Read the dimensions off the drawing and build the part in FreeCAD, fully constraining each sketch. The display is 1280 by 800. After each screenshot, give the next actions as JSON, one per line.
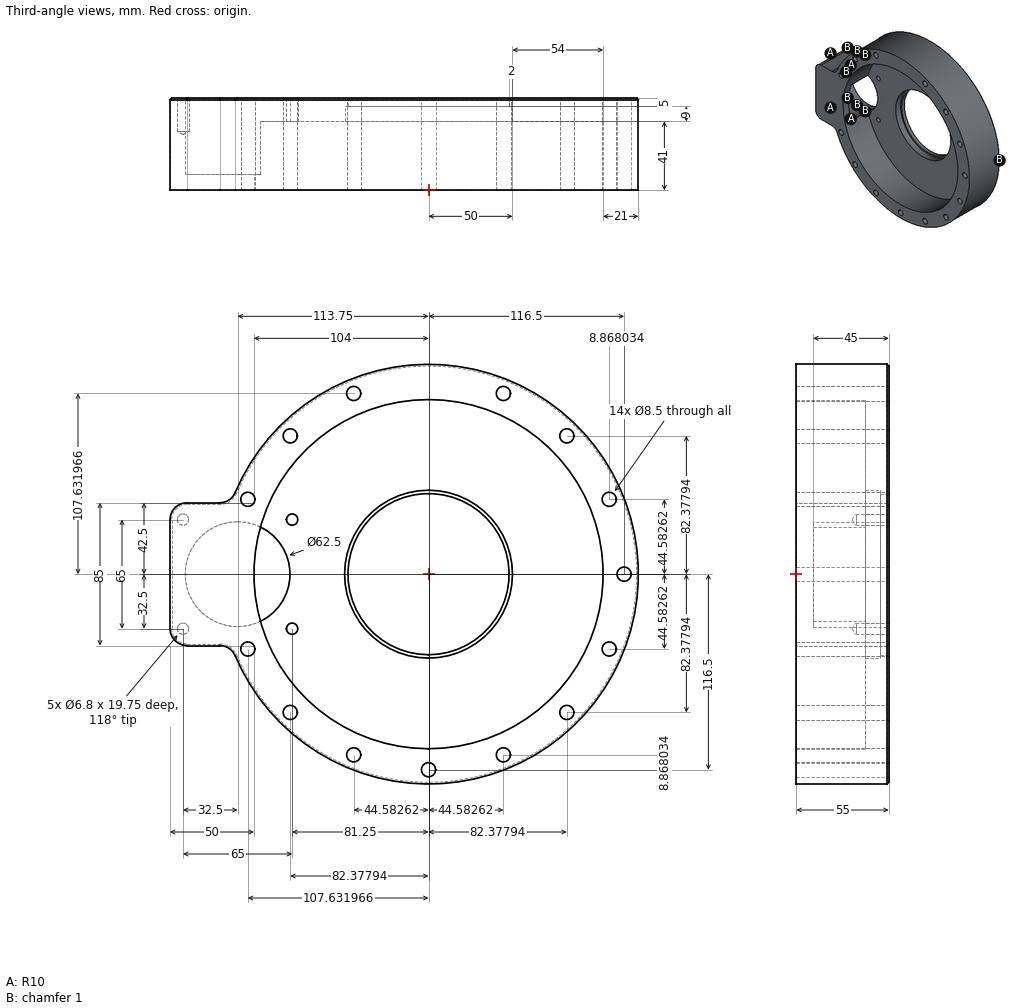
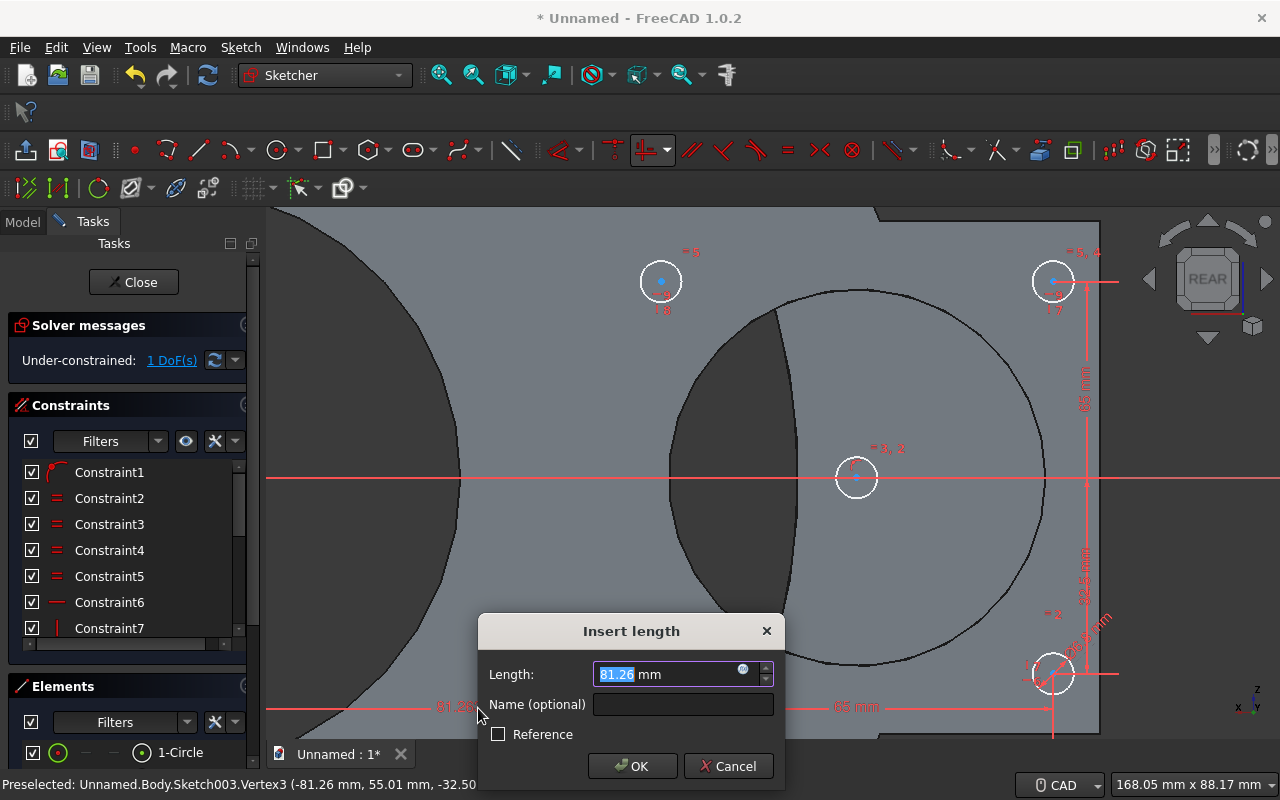
{"action": "type", "text": "81.25"}
{"action": "key", "text": "Return"}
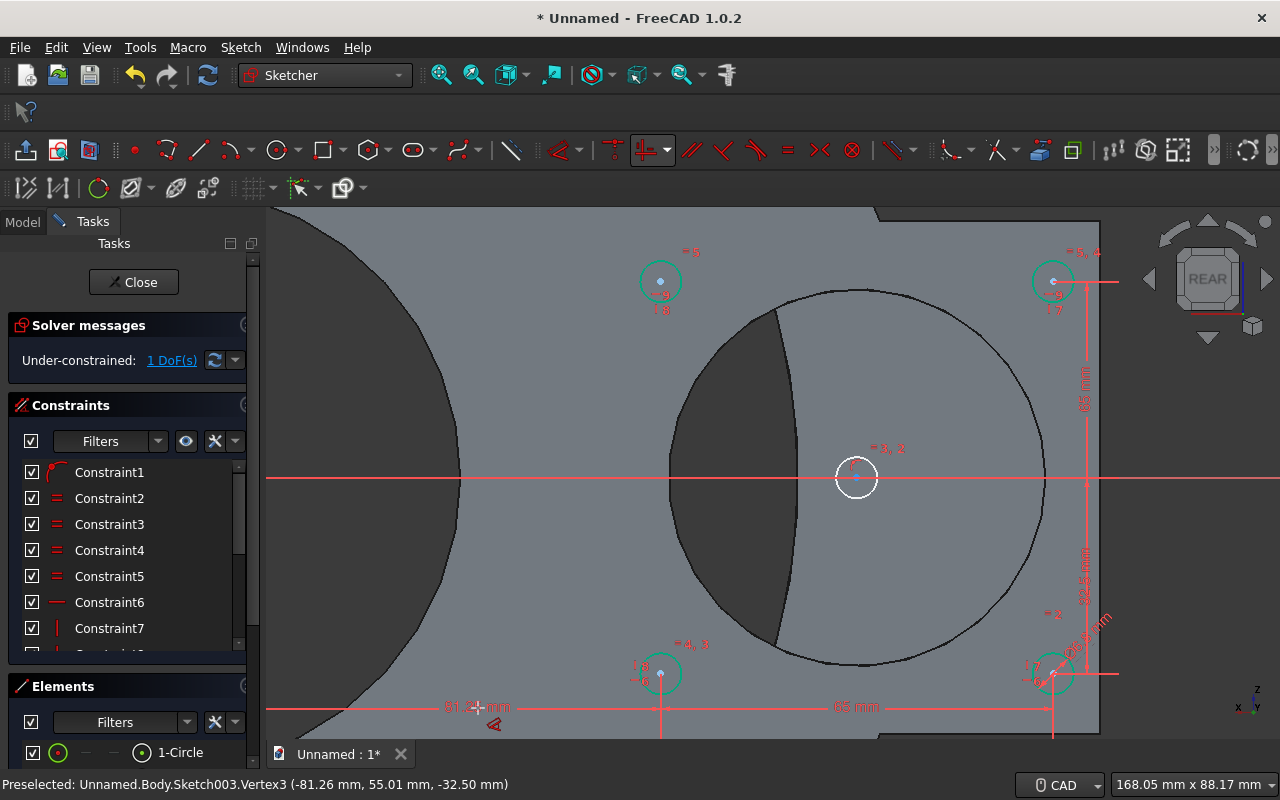
{"action": "left_click", "coordinate": [1053, 674]}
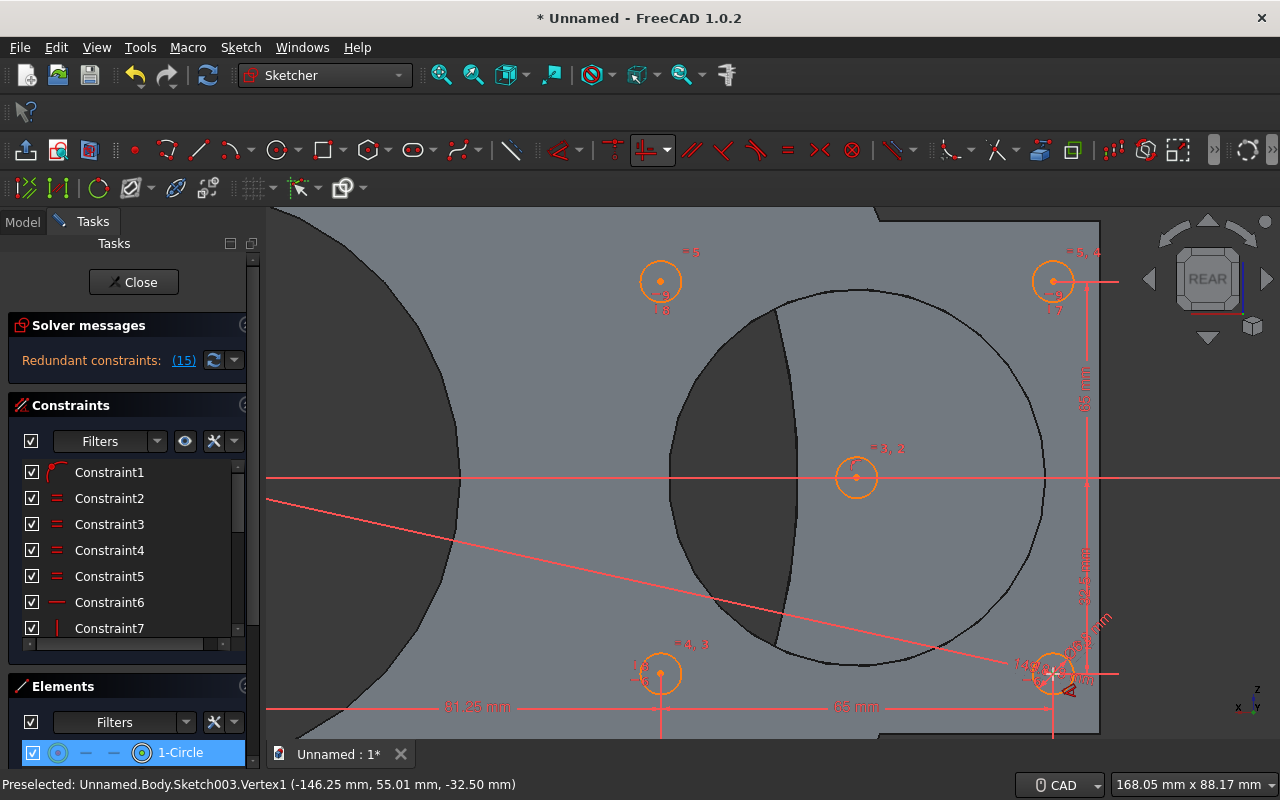
{"action": "left_click", "coordinate": [857, 478]}
{"action": "left_click", "coordinate": [955, 708]}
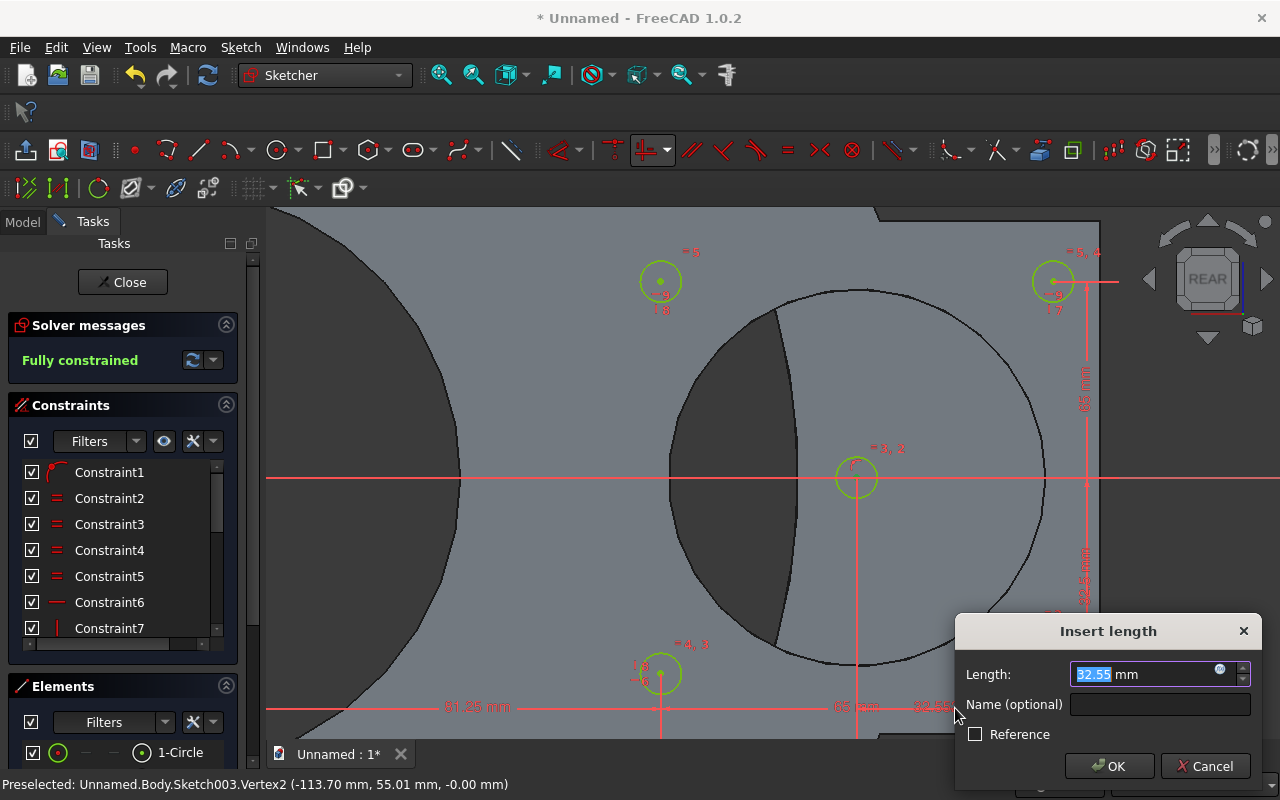
{"action": "type", "text": "32.5"}
{"action": "key", "text": "Return"}
{"action": "key", "text": "Escape"}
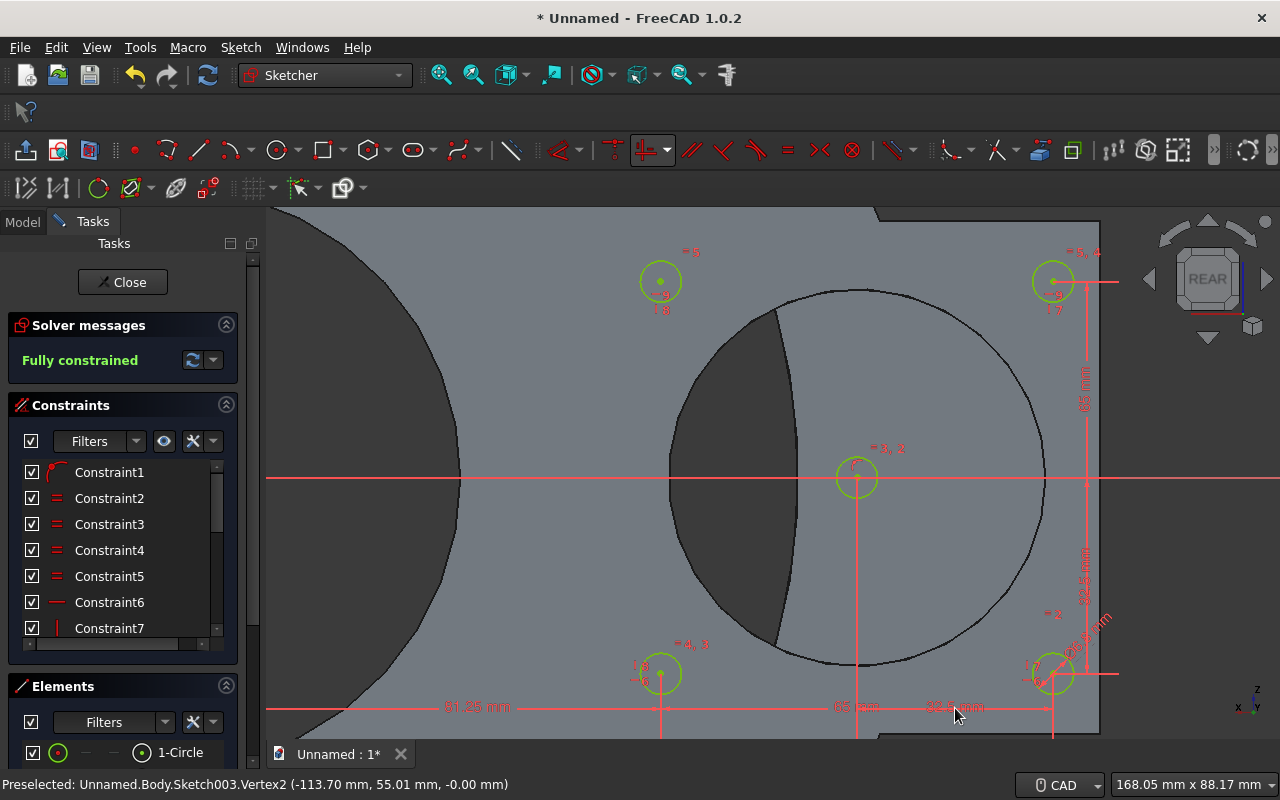
{"action": "left_click", "coordinate": [123, 282]}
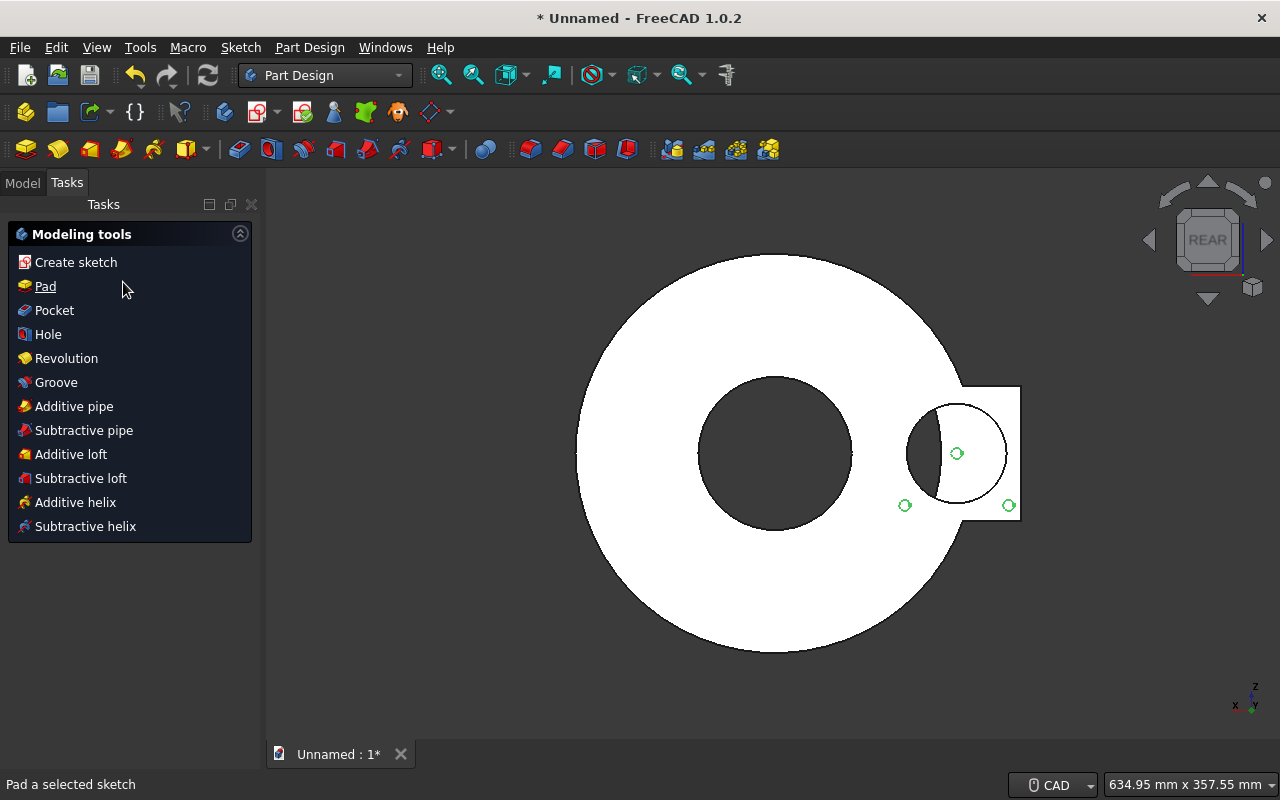
{"action": "left_click", "coordinate": [272, 150]}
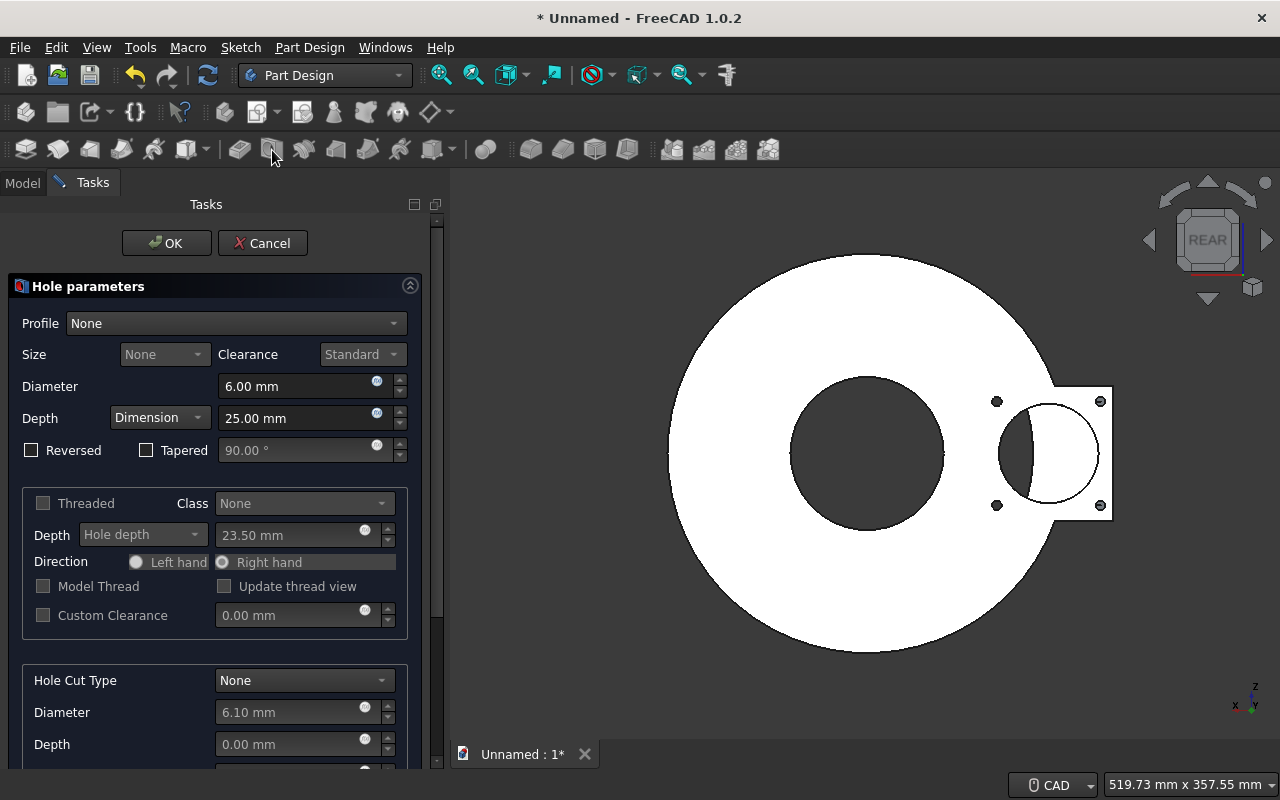
{"action": "triple_click", "coordinate": [305, 386]}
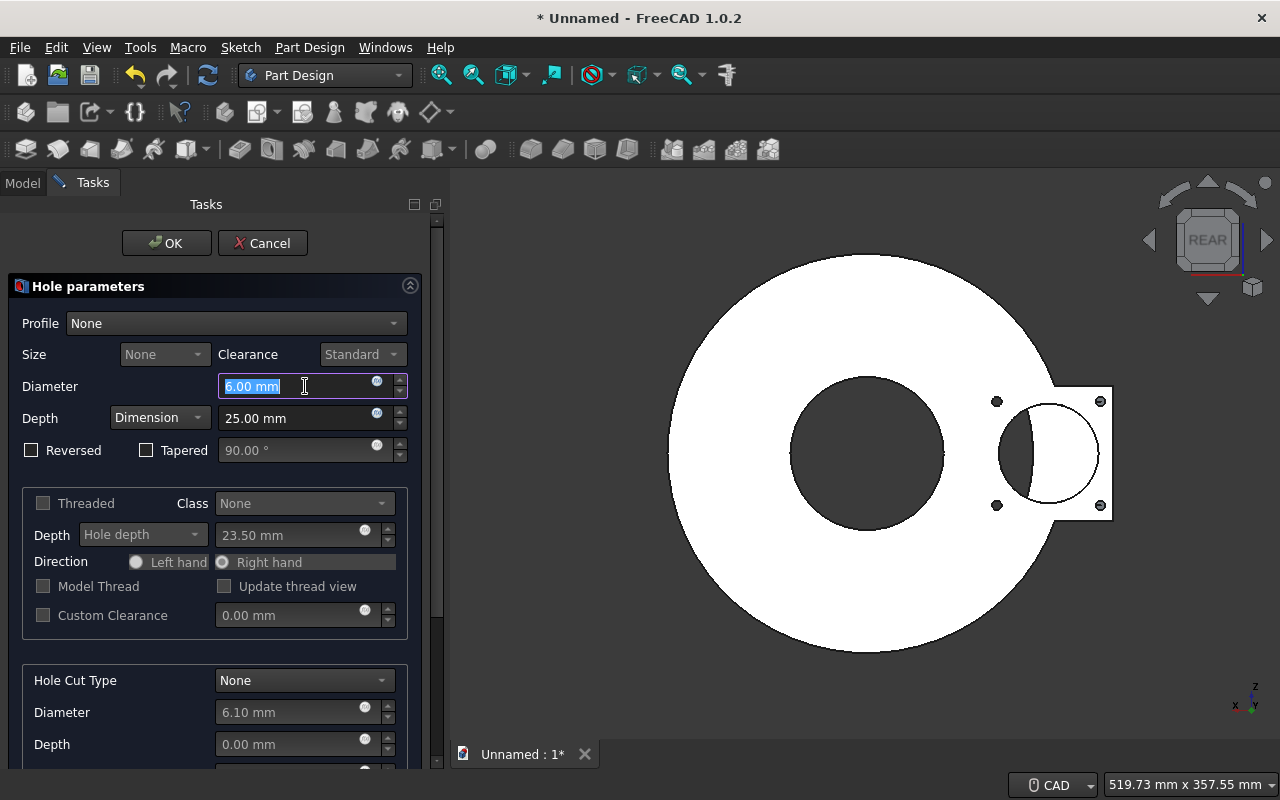
{"action": "type", "text": "6.8"}
{"action": "key", "text": "Tab"}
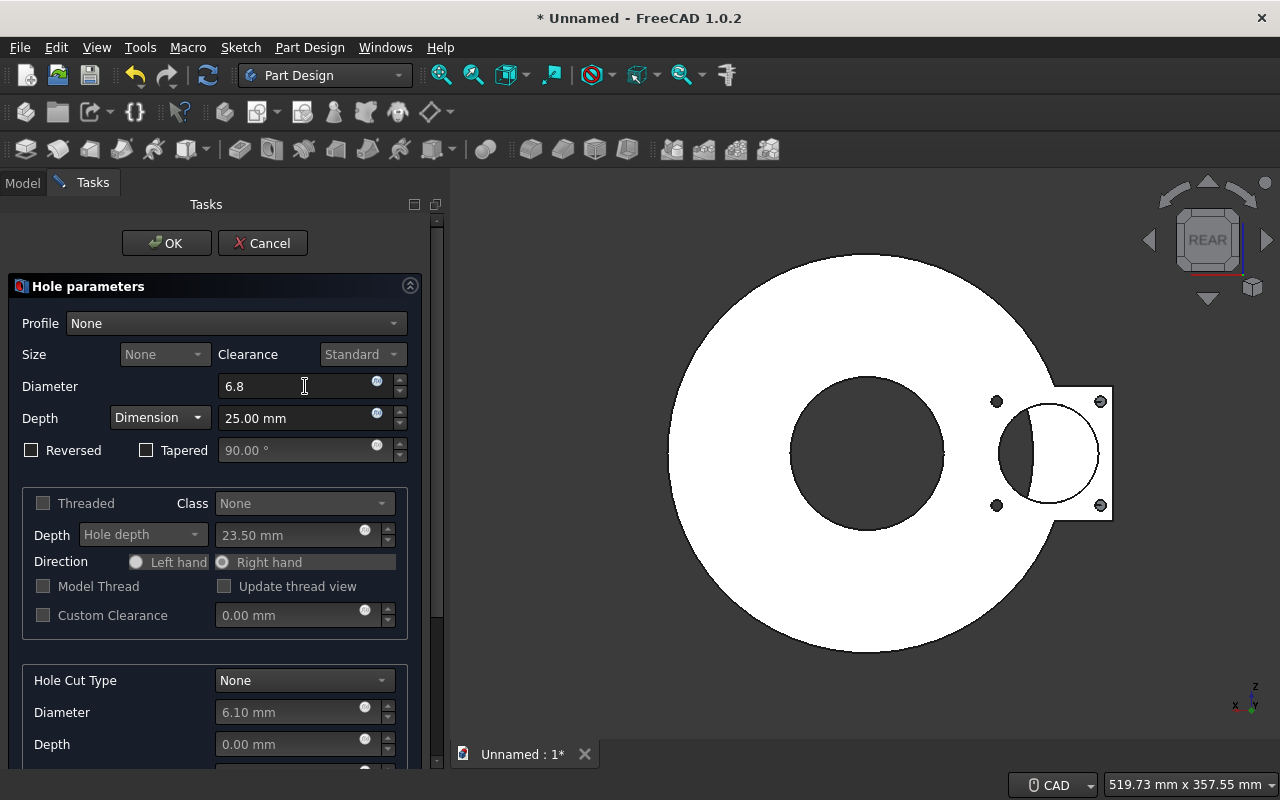
{"action": "triple_click", "coordinate": [305, 418]}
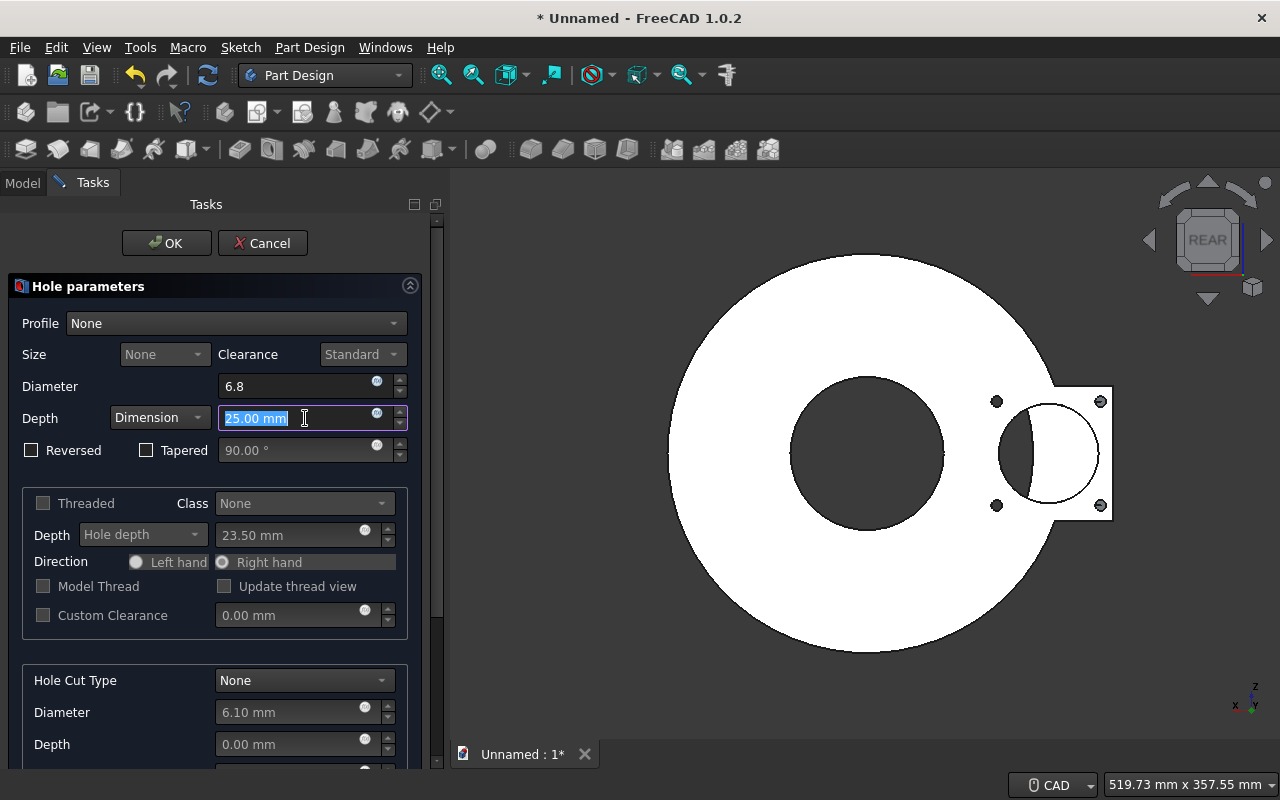
{"action": "type", "text": "19.75"}
{"action": "key", "text": "Tab"}